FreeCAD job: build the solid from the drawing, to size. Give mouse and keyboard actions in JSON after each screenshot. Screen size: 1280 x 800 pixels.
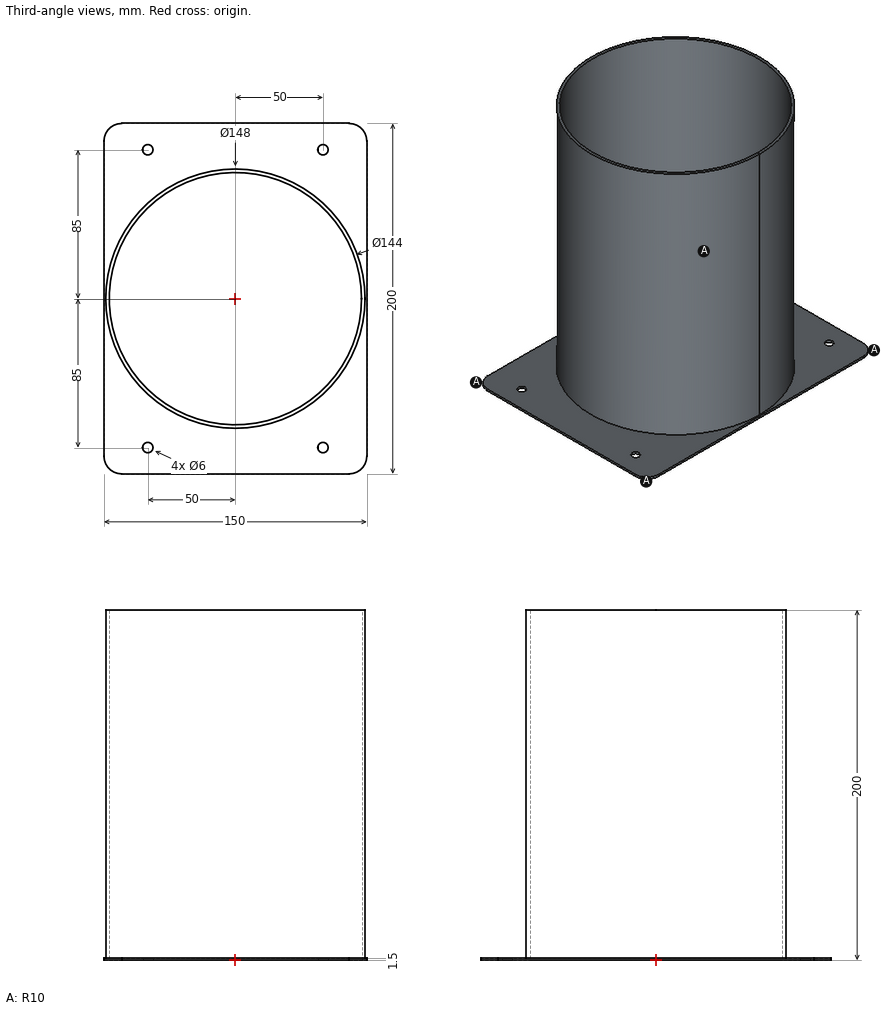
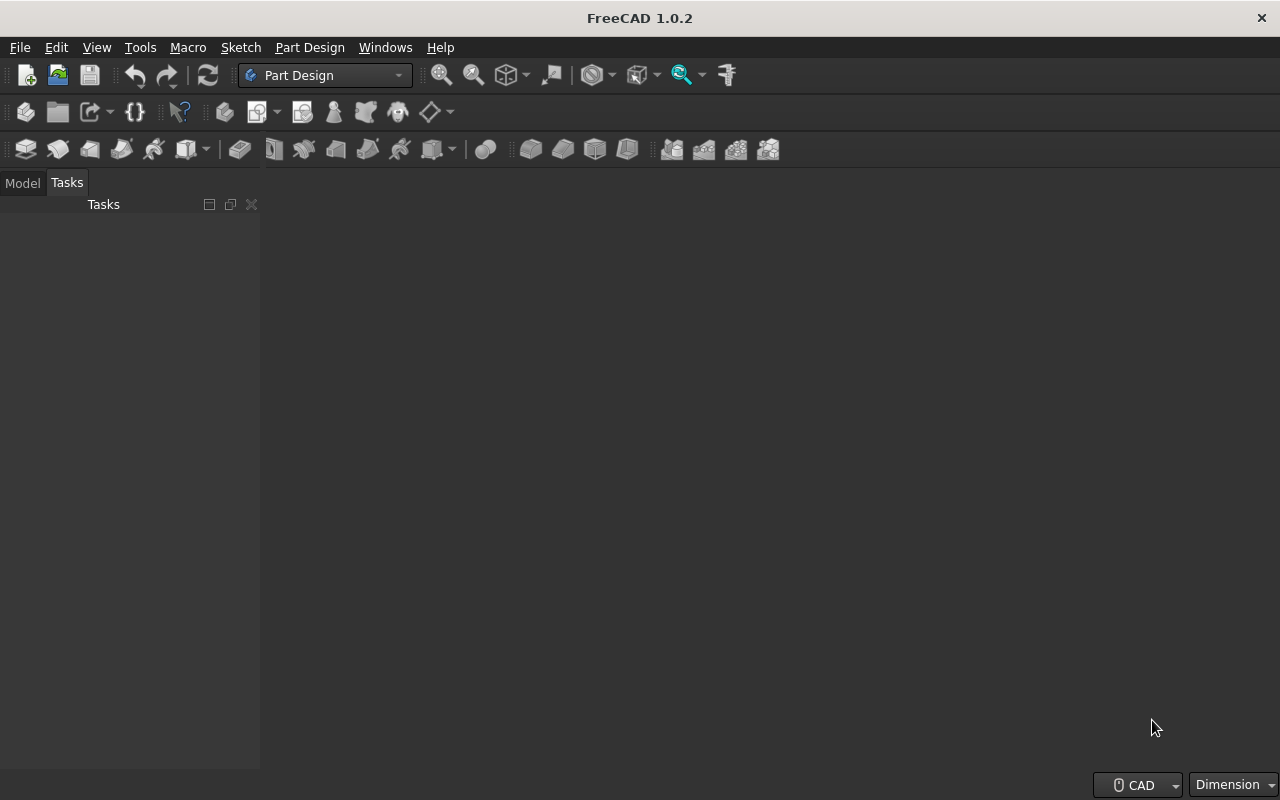
{"action": "left_click", "coordinate": [26, 76]}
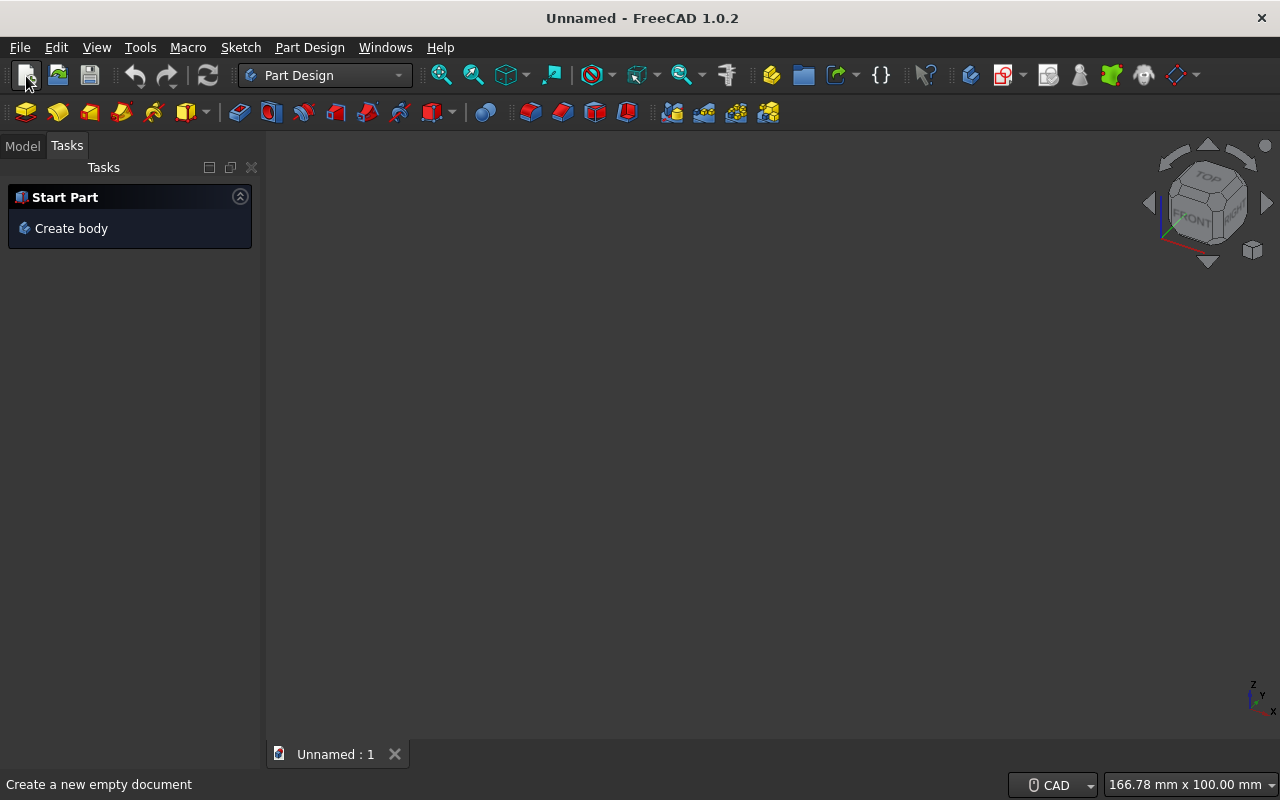
{"action": "left_click", "coordinate": [1004, 76]}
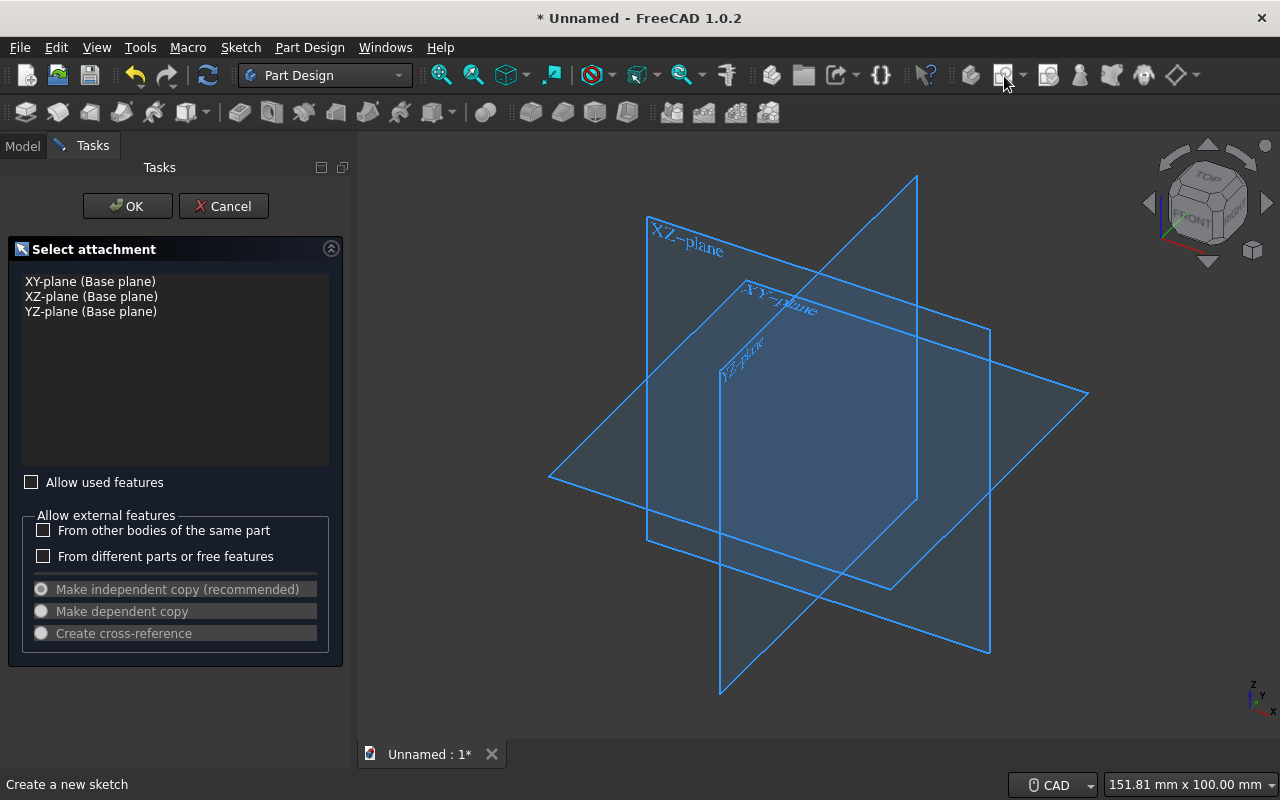
{"action": "left_click", "coordinate": [82, 282]}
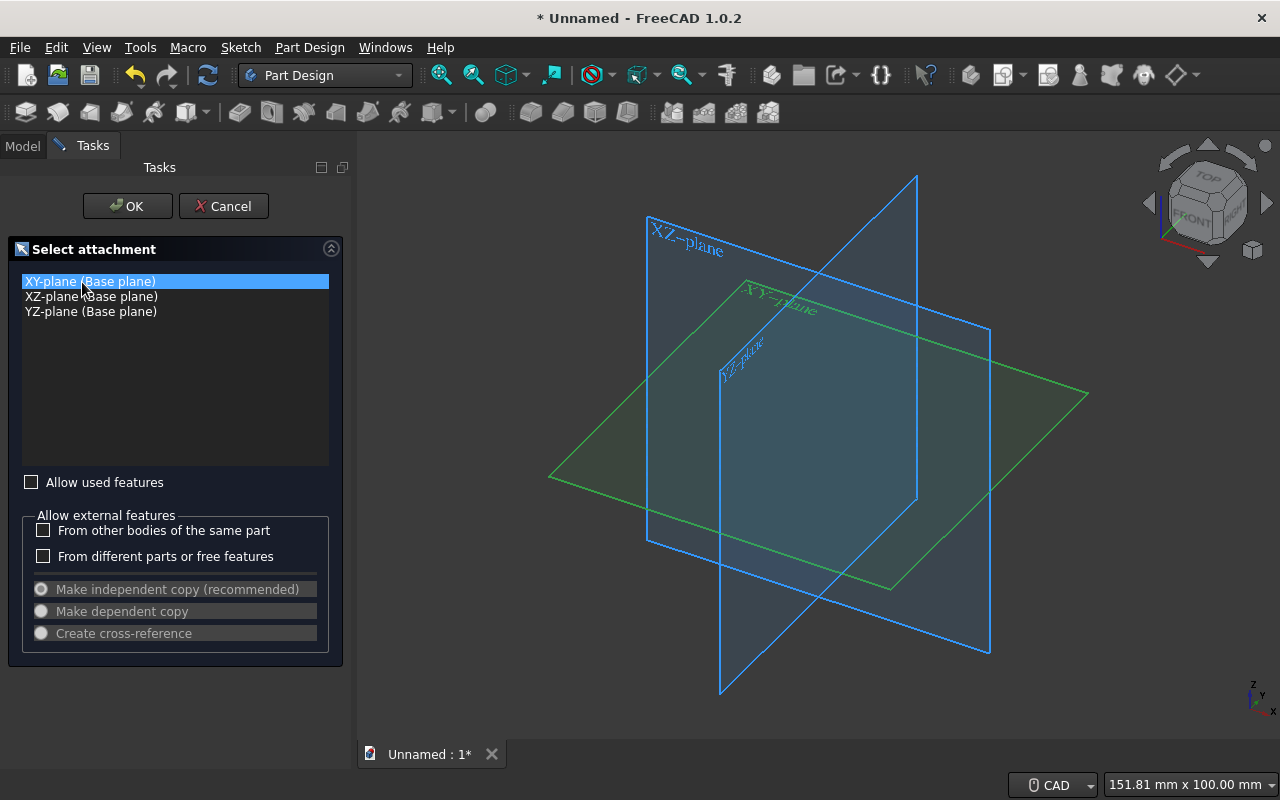
{"action": "left_click", "coordinate": [128, 206]}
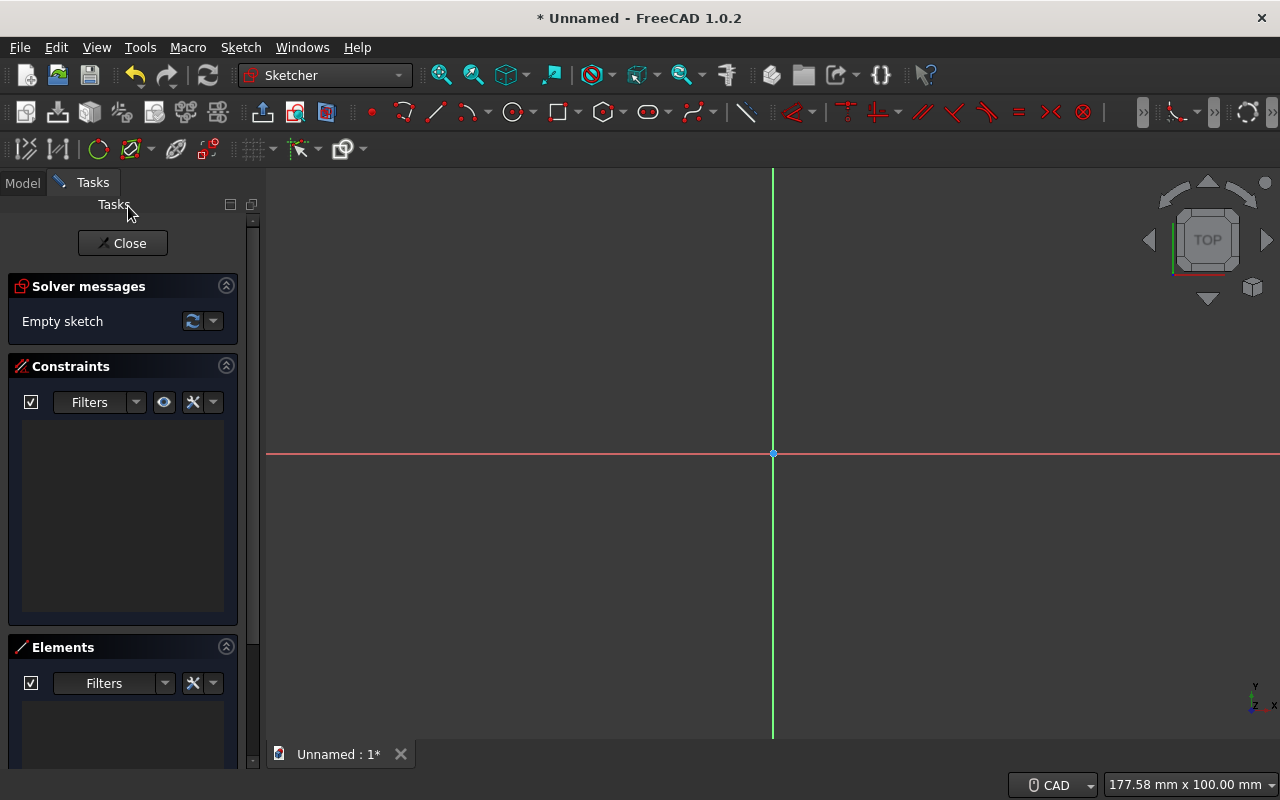
{"action": "scroll", "coordinate": [649, 454], "scroll_direction": "down", "scroll_amount": 4}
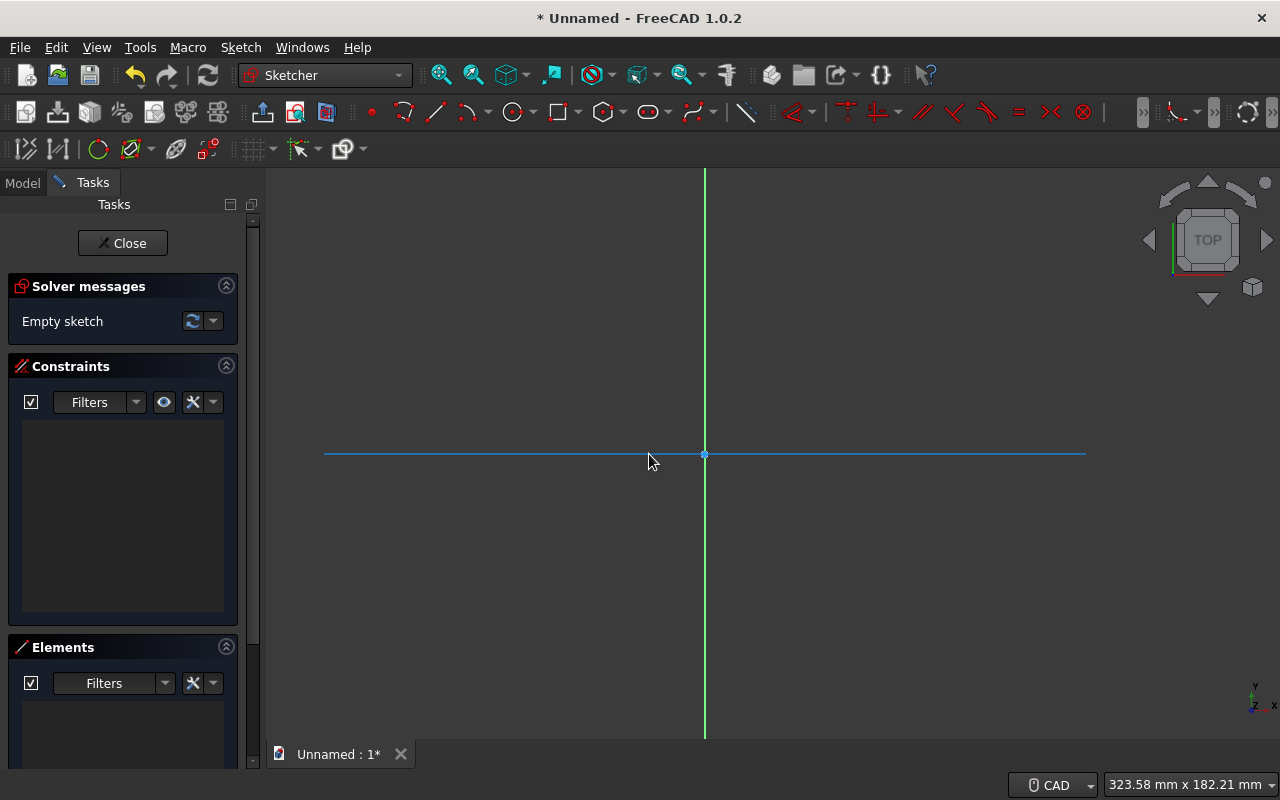
{"action": "left_click", "coordinate": [514, 112]}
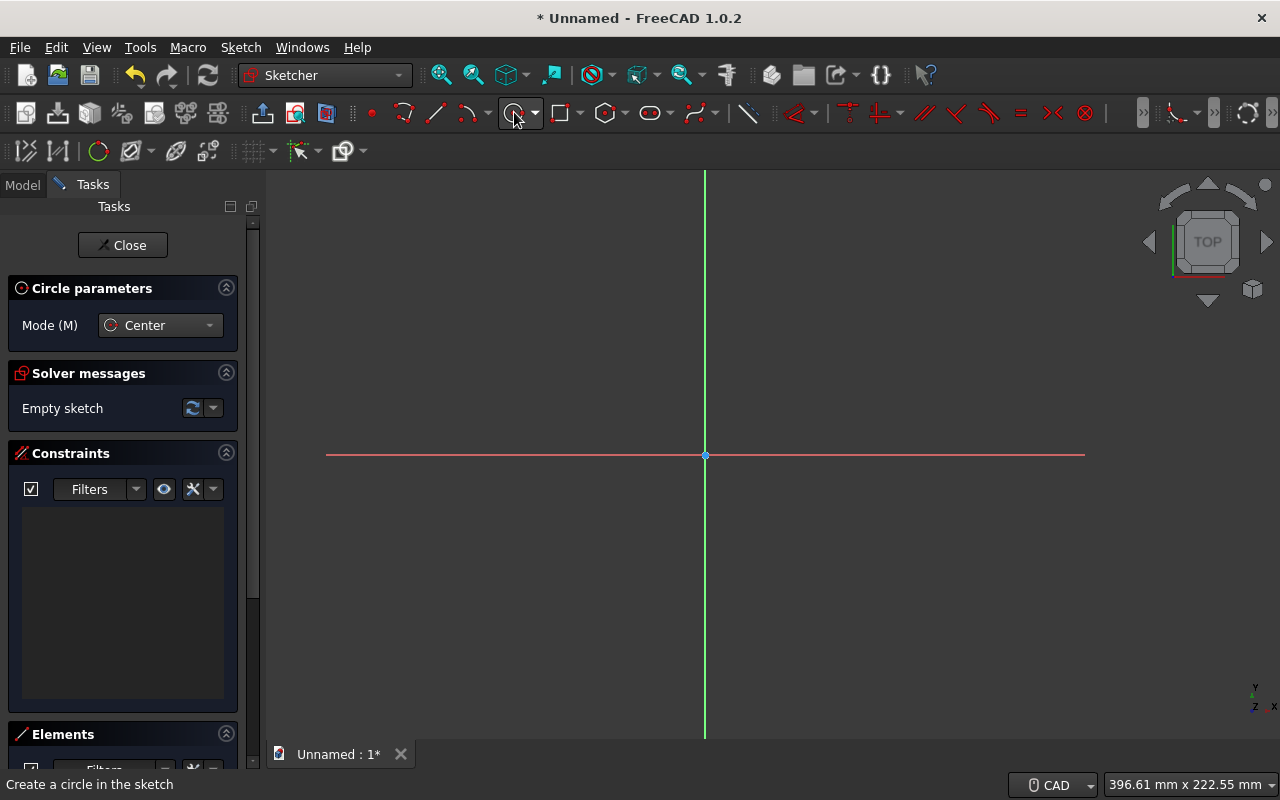
{"action": "left_click", "coordinate": [705, 455]}
{"action": "mouse_move", "coordinate": [839, 321]}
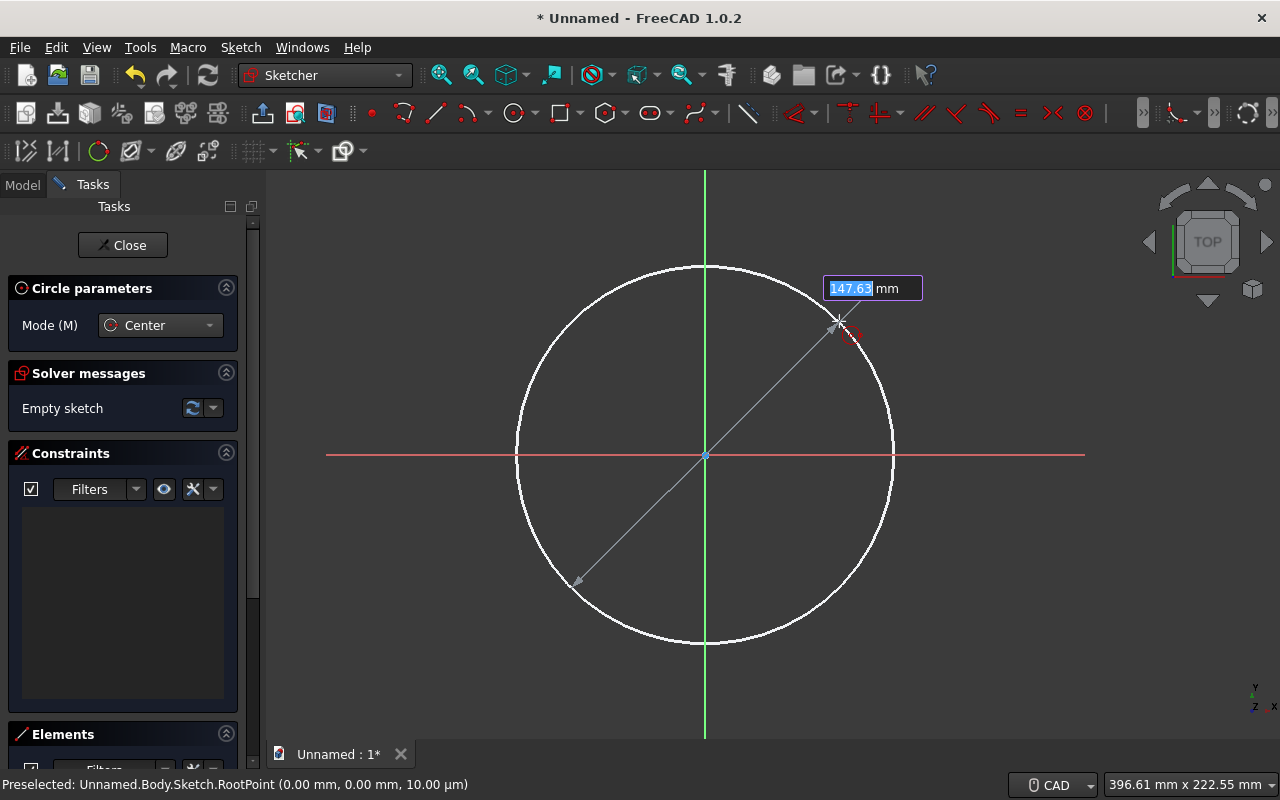
{"action": "type", "text": "148"}
{"action": "key", "text": "Return"}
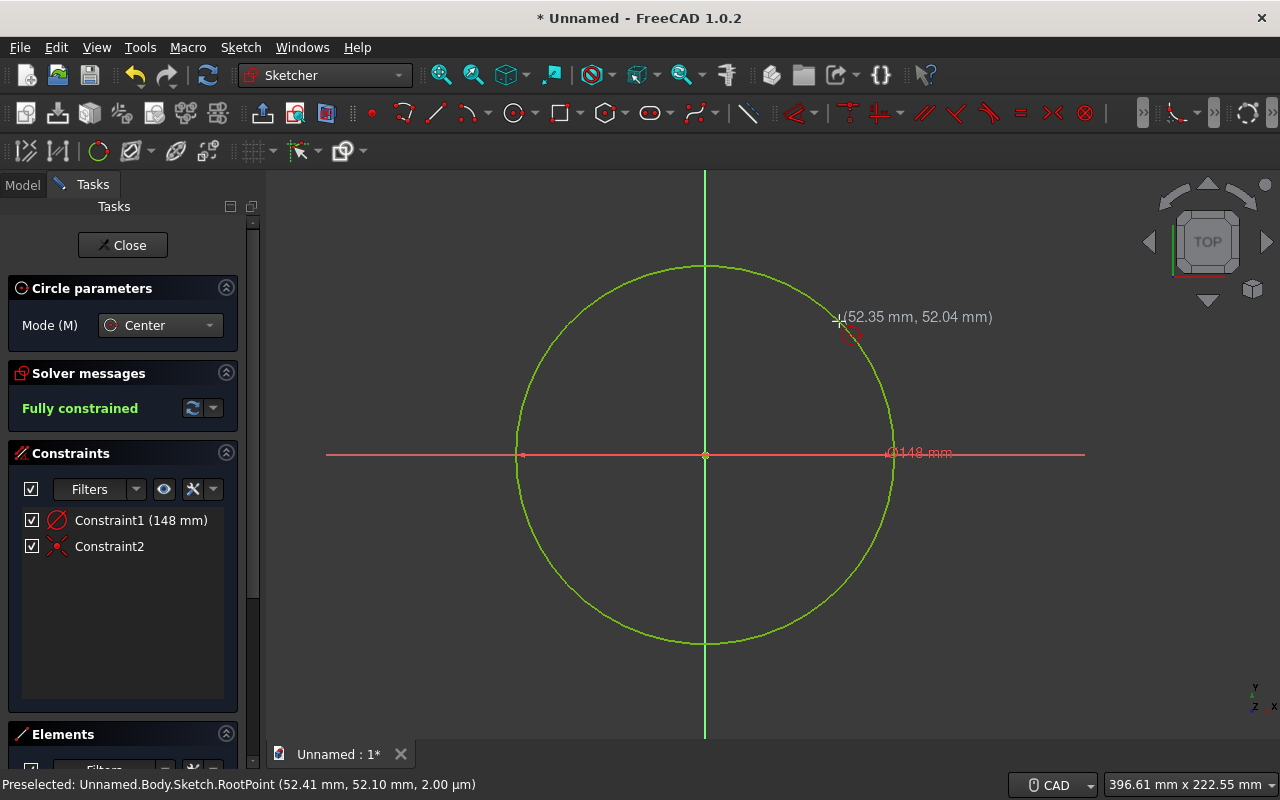
{"action": "left_click", "coordinate": [705, 455]}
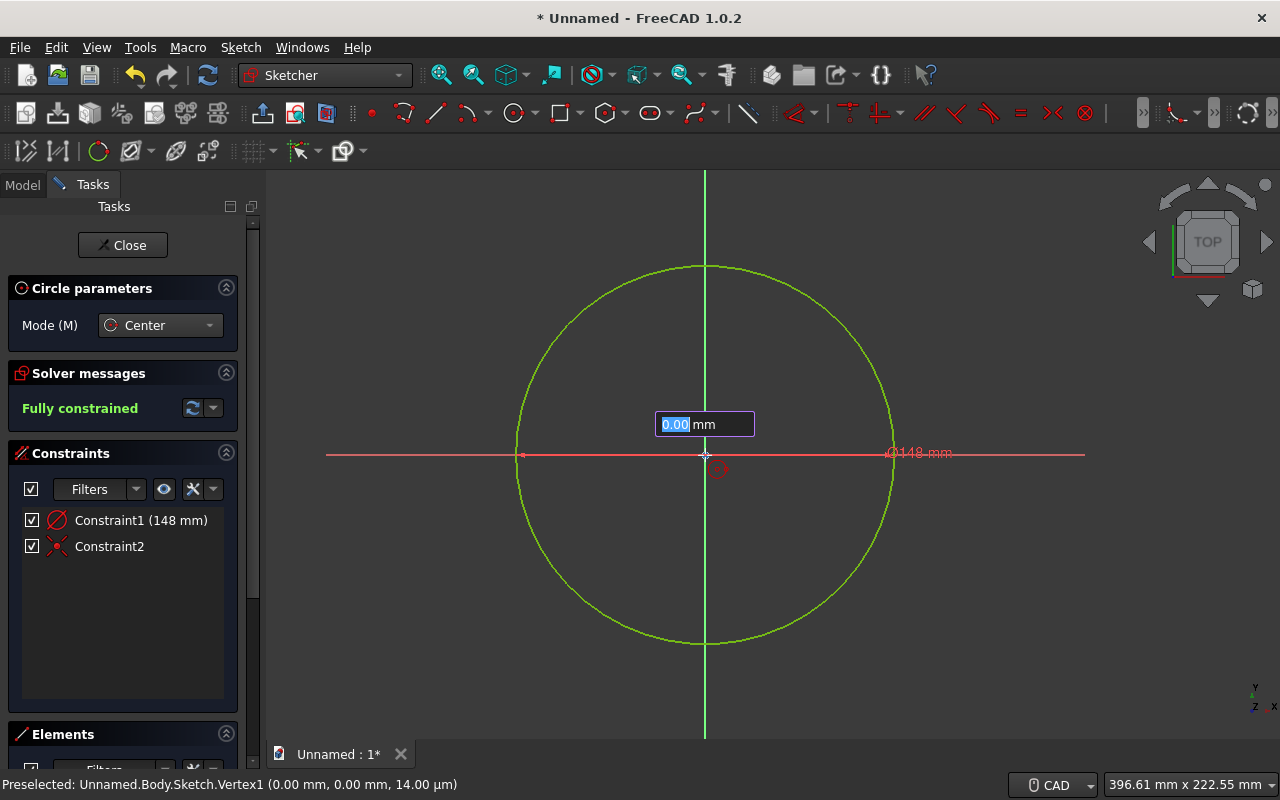
{"action": "scroll", "coordinate": [835, 325], "scroll_direction": "up", "scroll_amount": 6}
{"action": "mouse_move", "coordinate": [835, 324]}